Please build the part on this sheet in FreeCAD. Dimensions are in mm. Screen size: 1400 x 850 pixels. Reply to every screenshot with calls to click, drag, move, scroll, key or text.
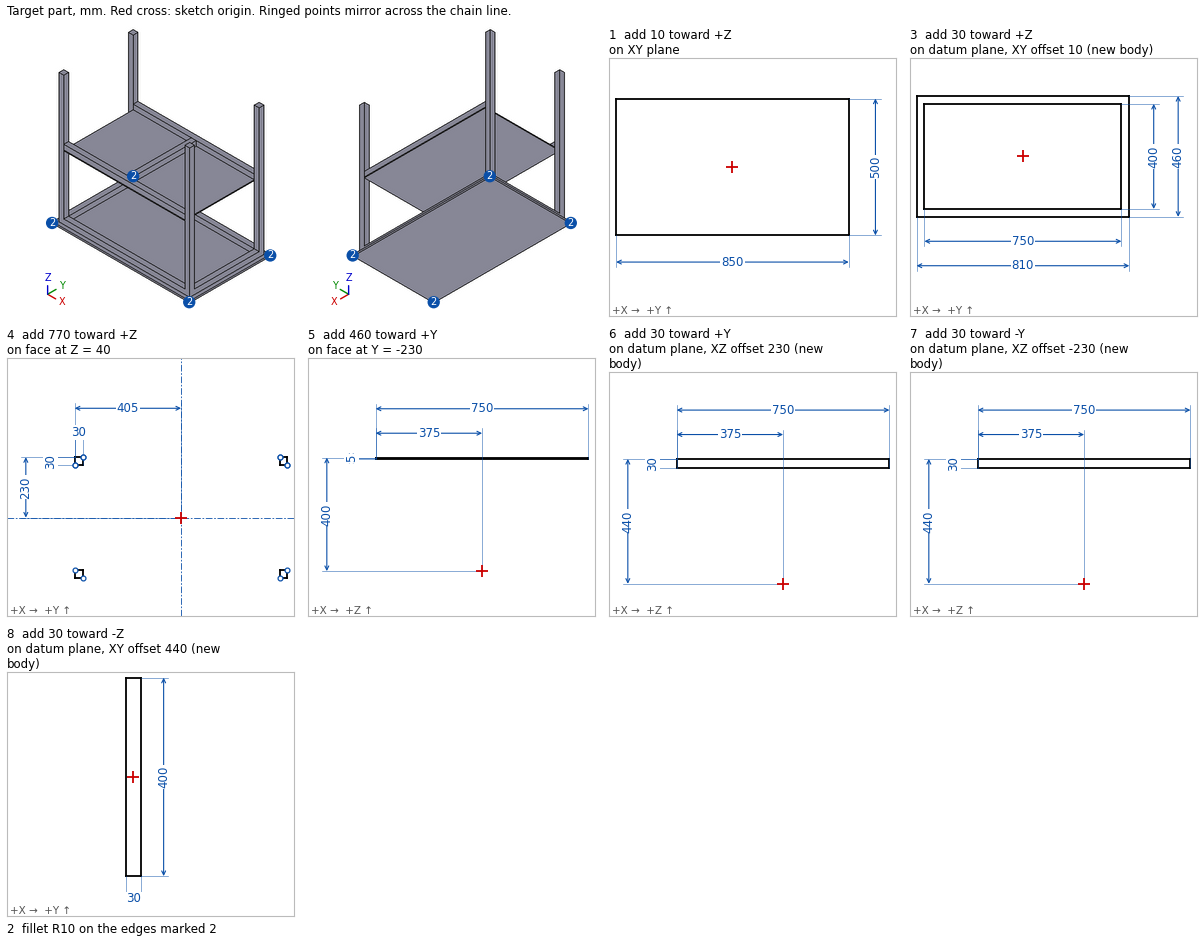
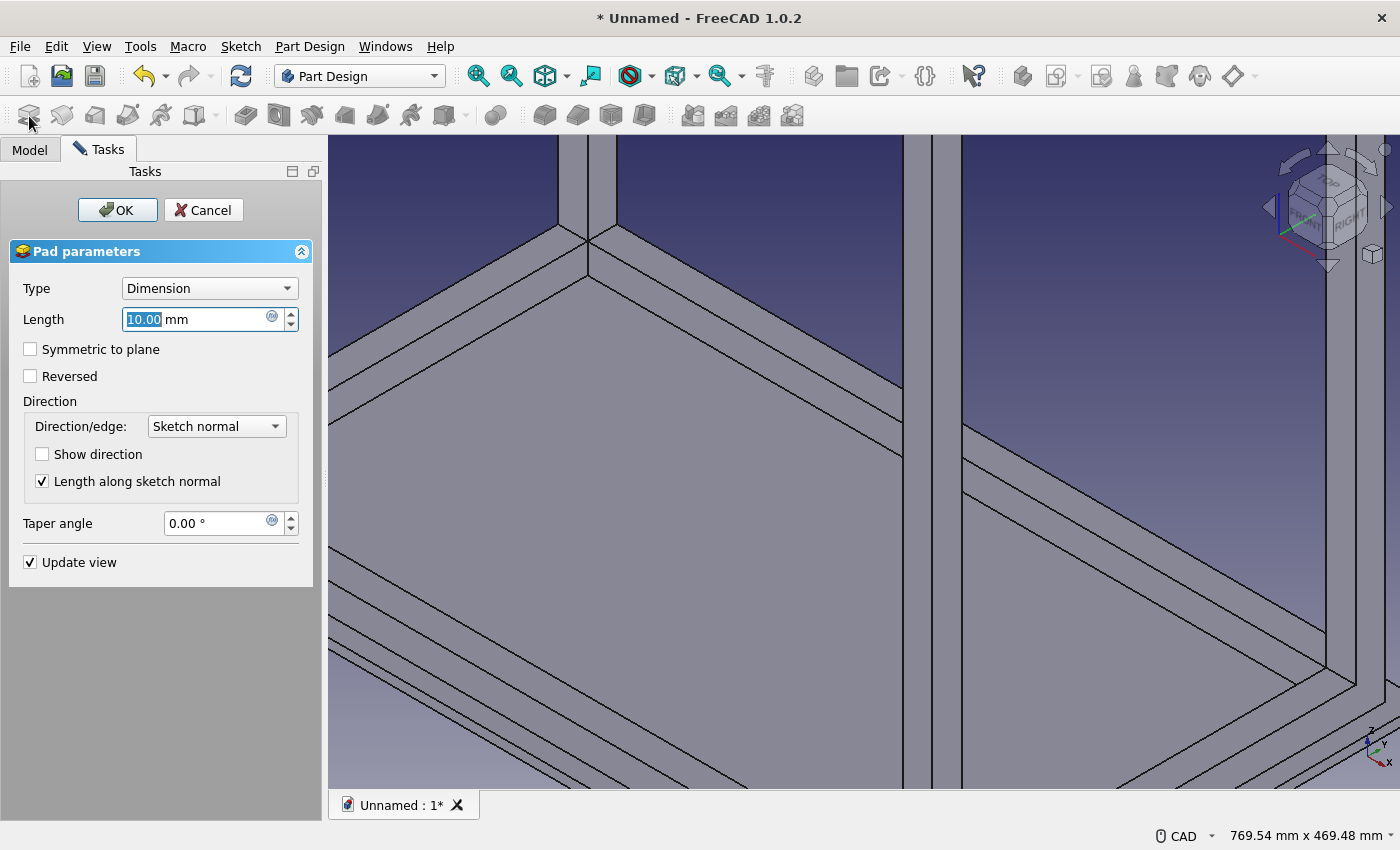
text(460)
key(Tab)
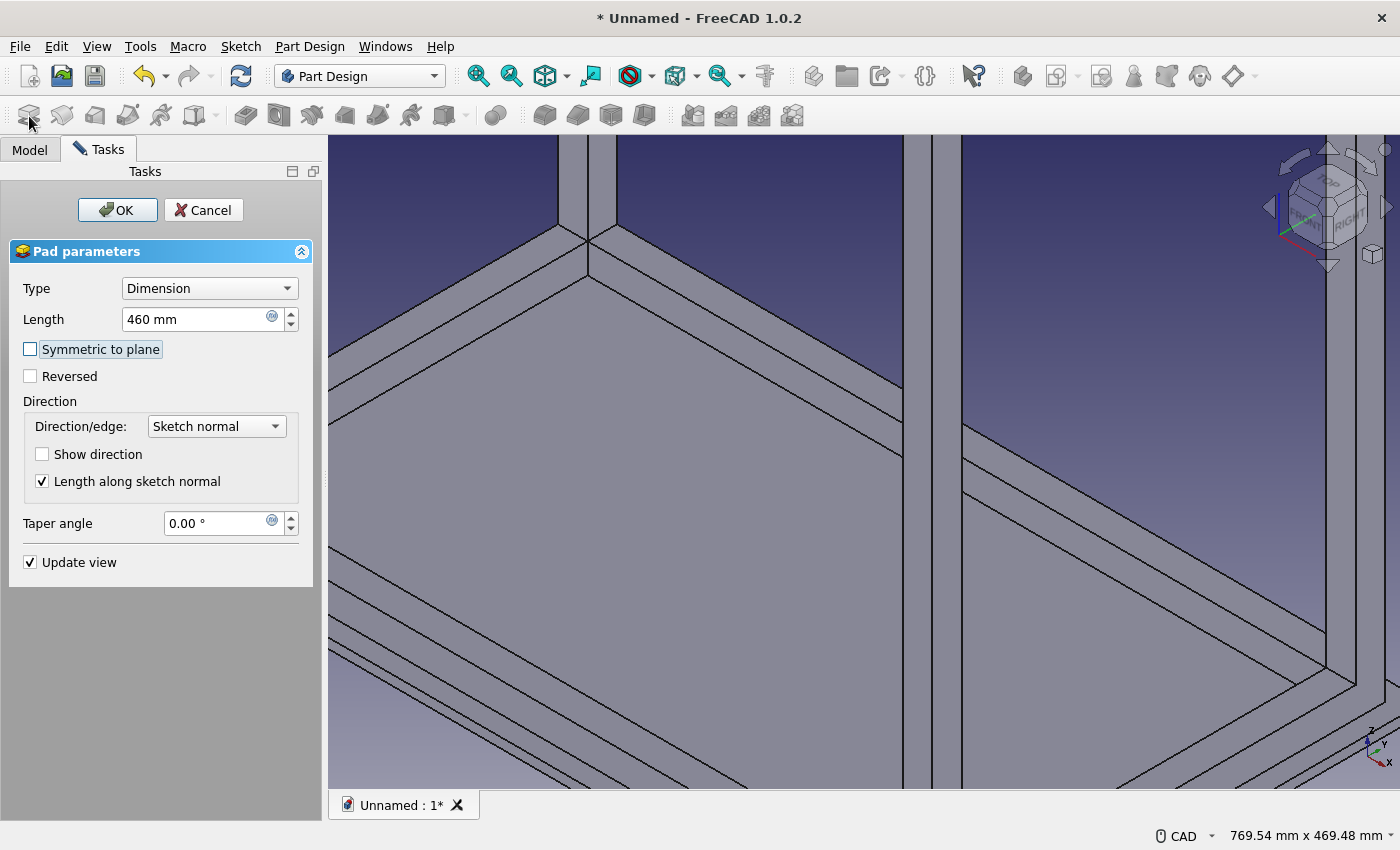
click(31, 376)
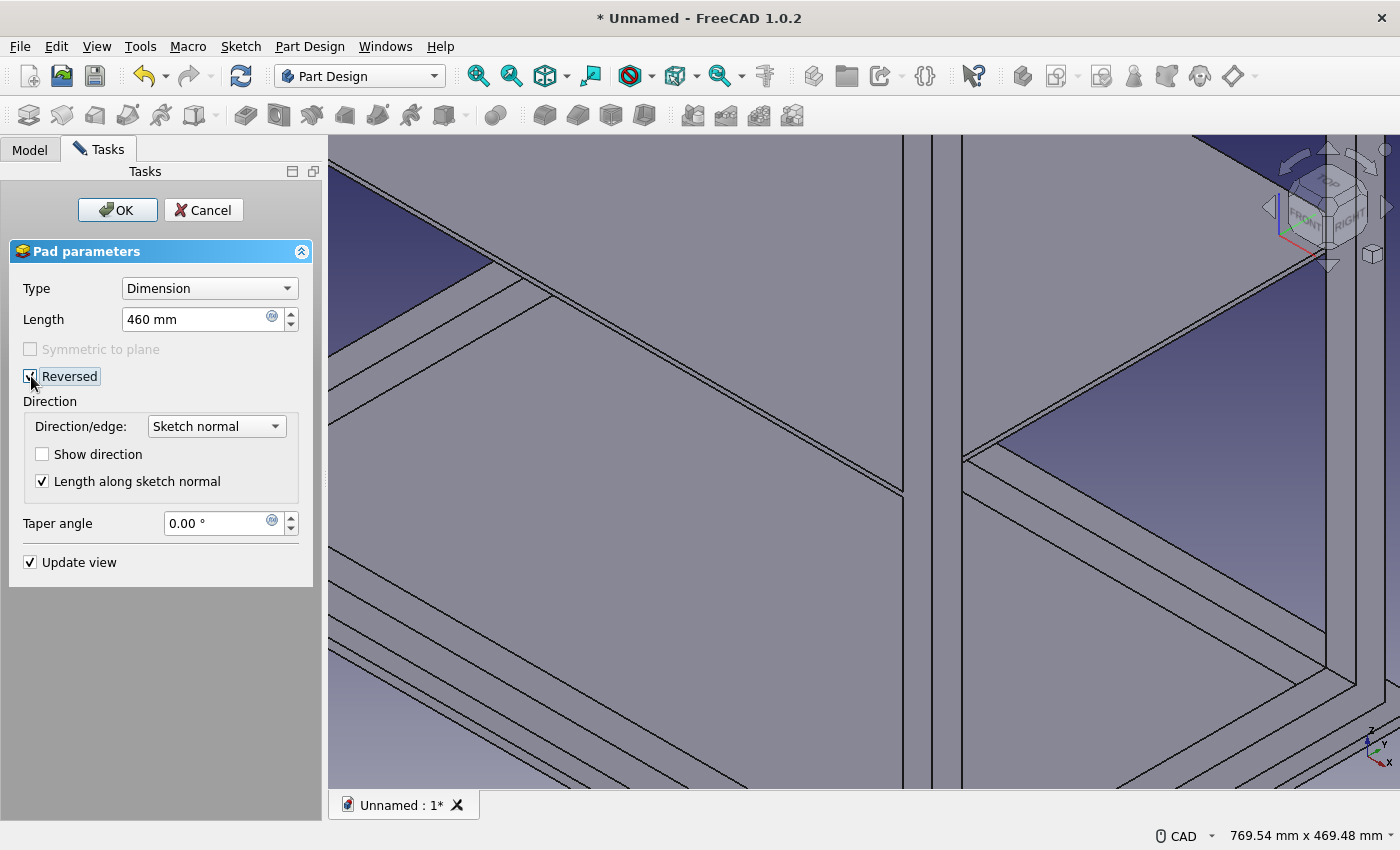
click(118, 210)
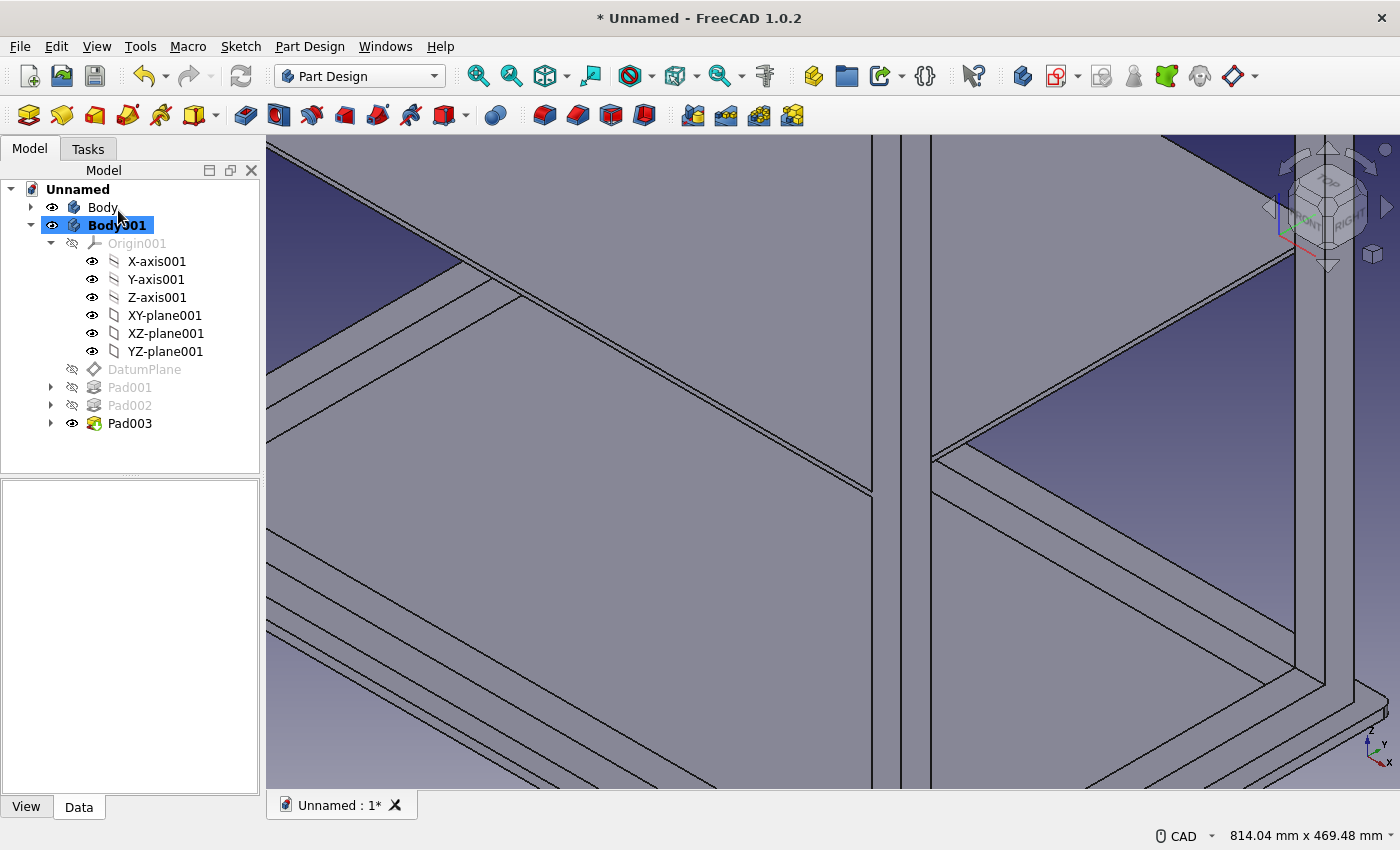
click(479, 76)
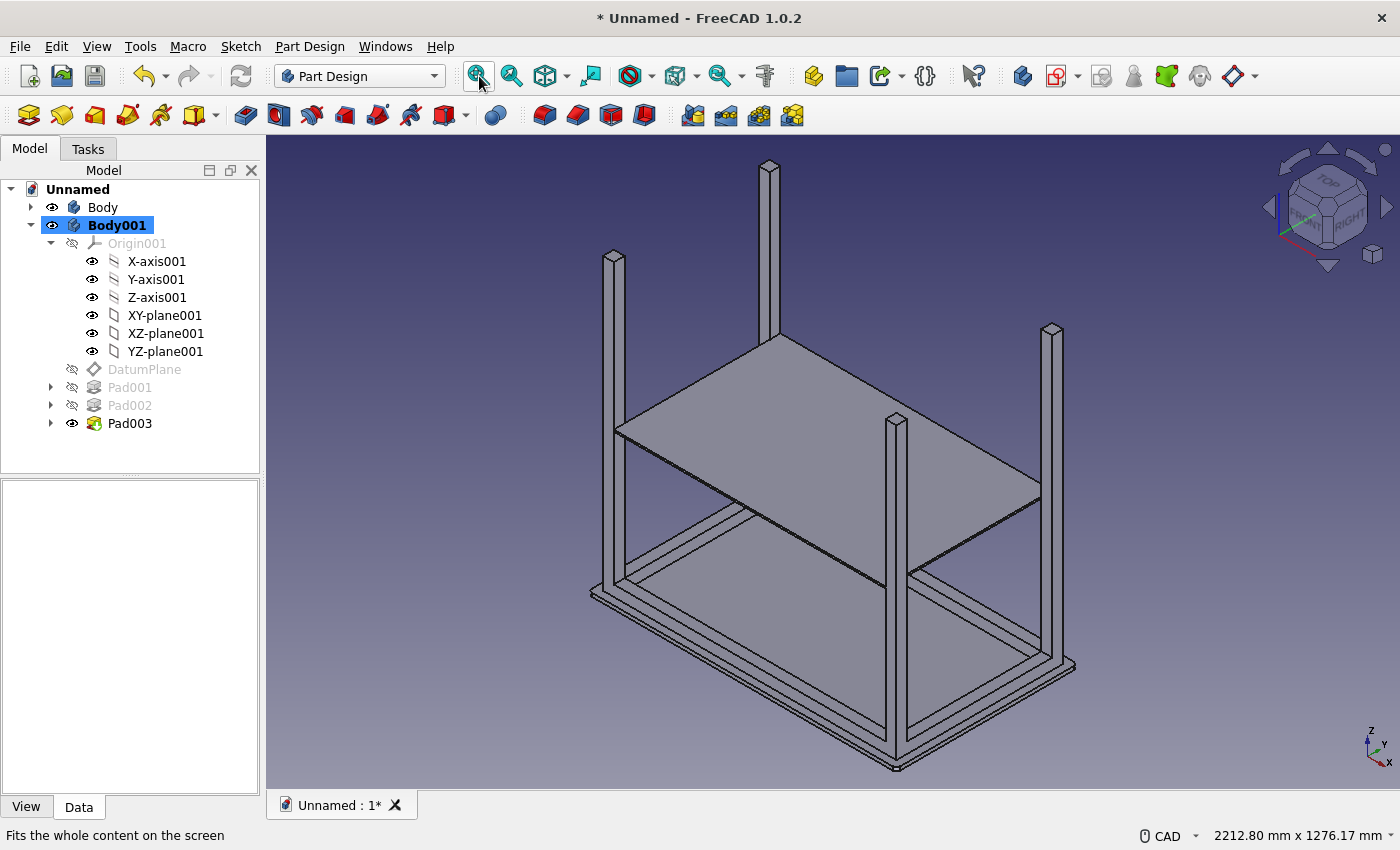
click(1023, 76)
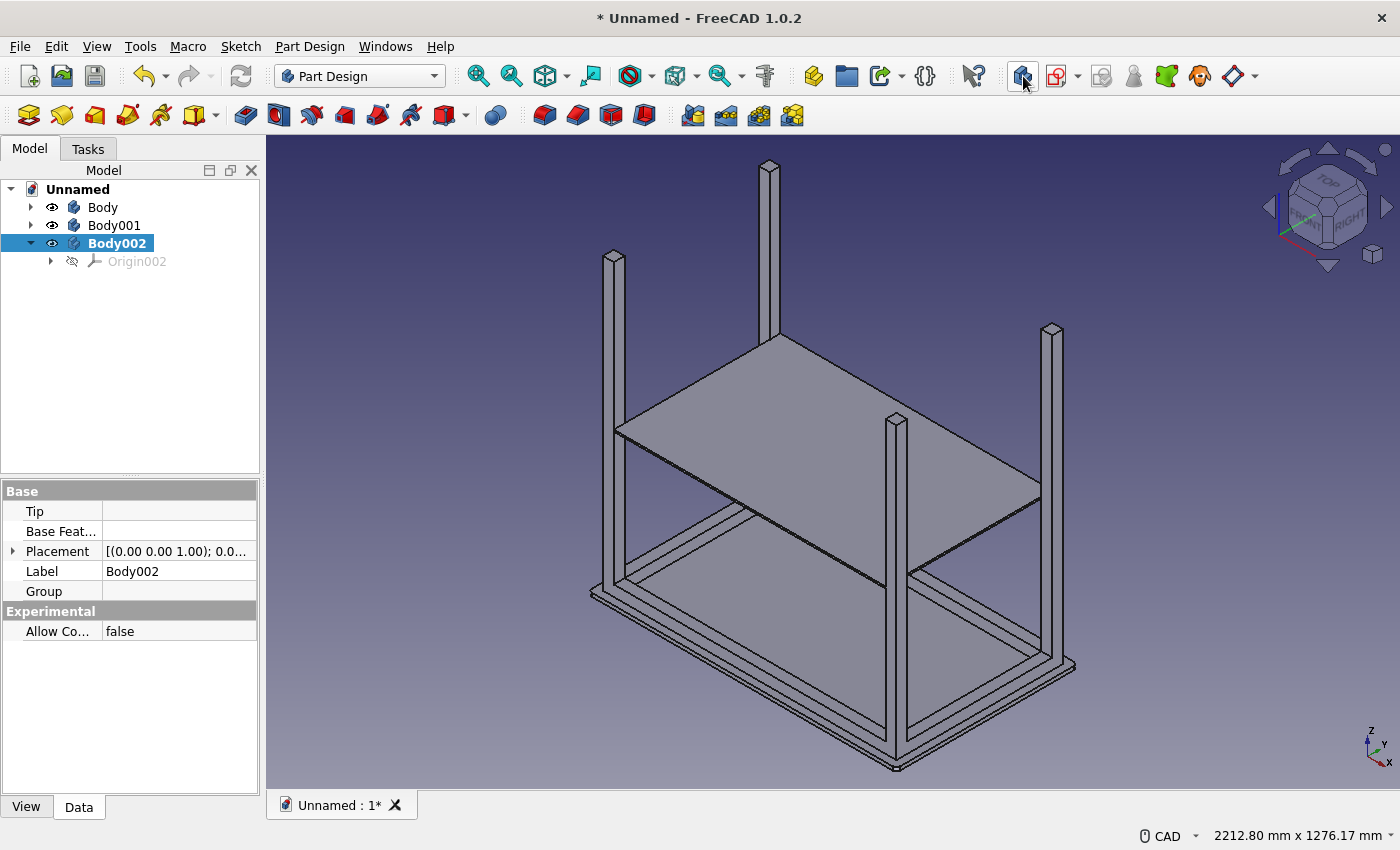
click(51, 261)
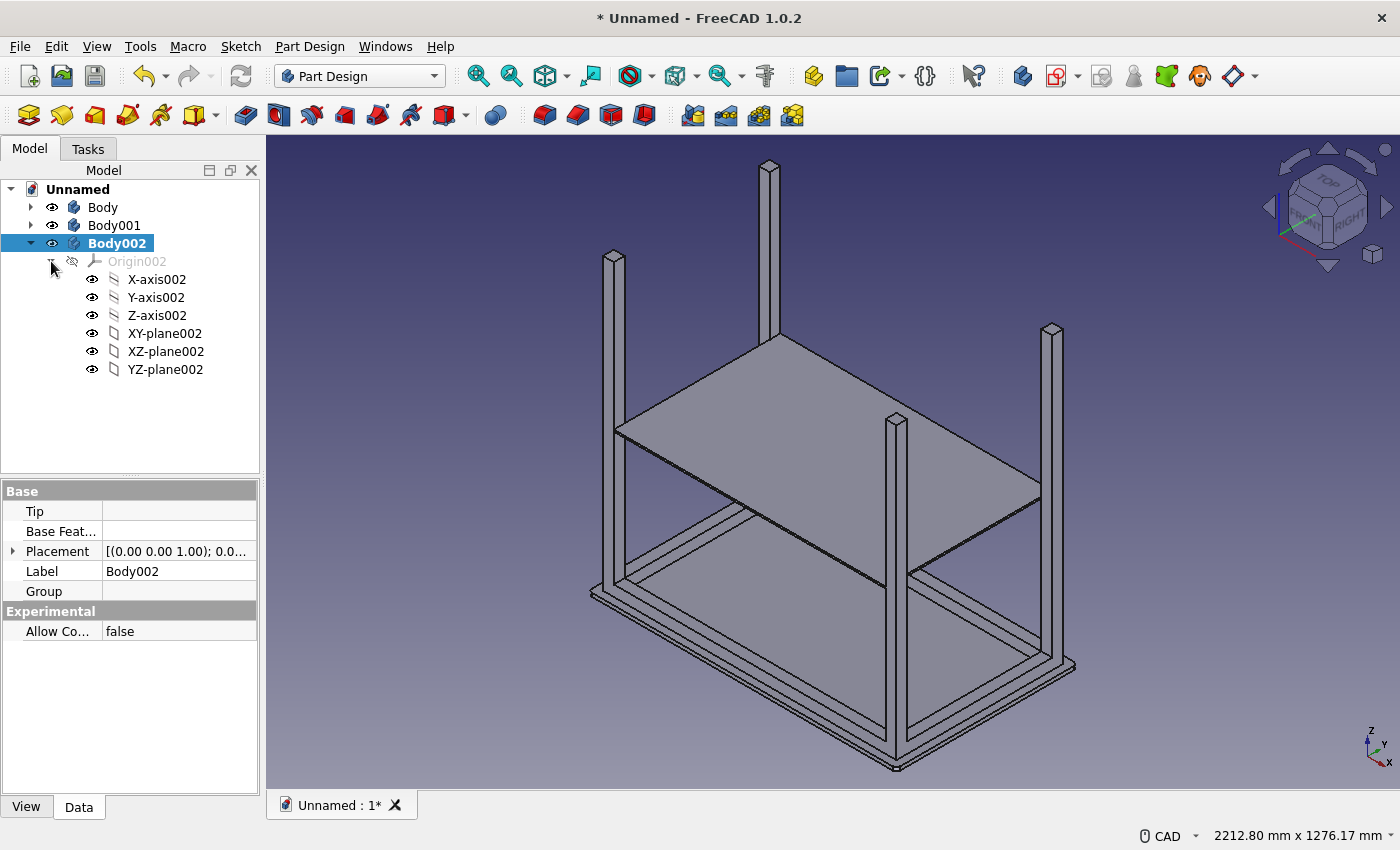
click(137, 351)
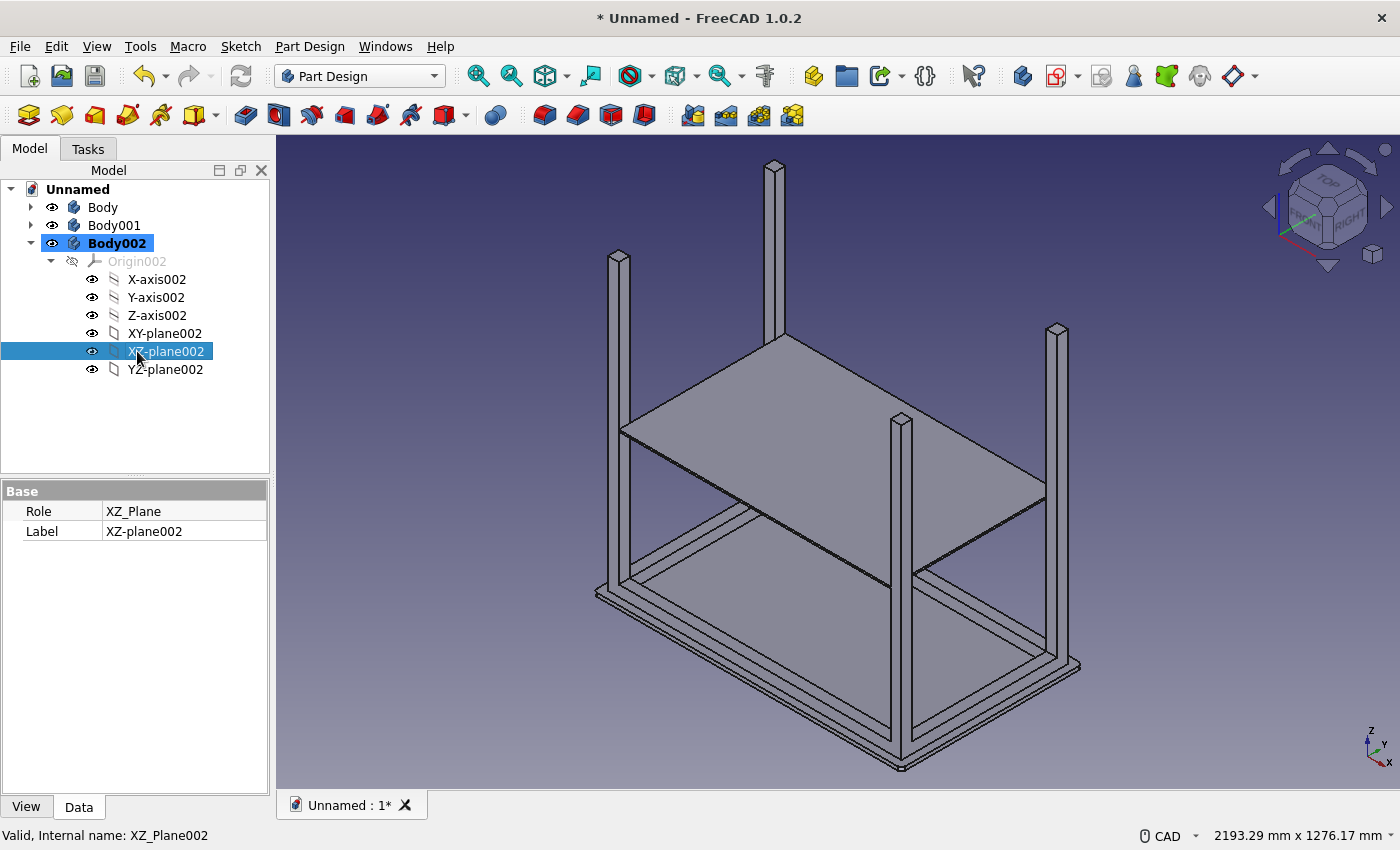
click(1232, 76)